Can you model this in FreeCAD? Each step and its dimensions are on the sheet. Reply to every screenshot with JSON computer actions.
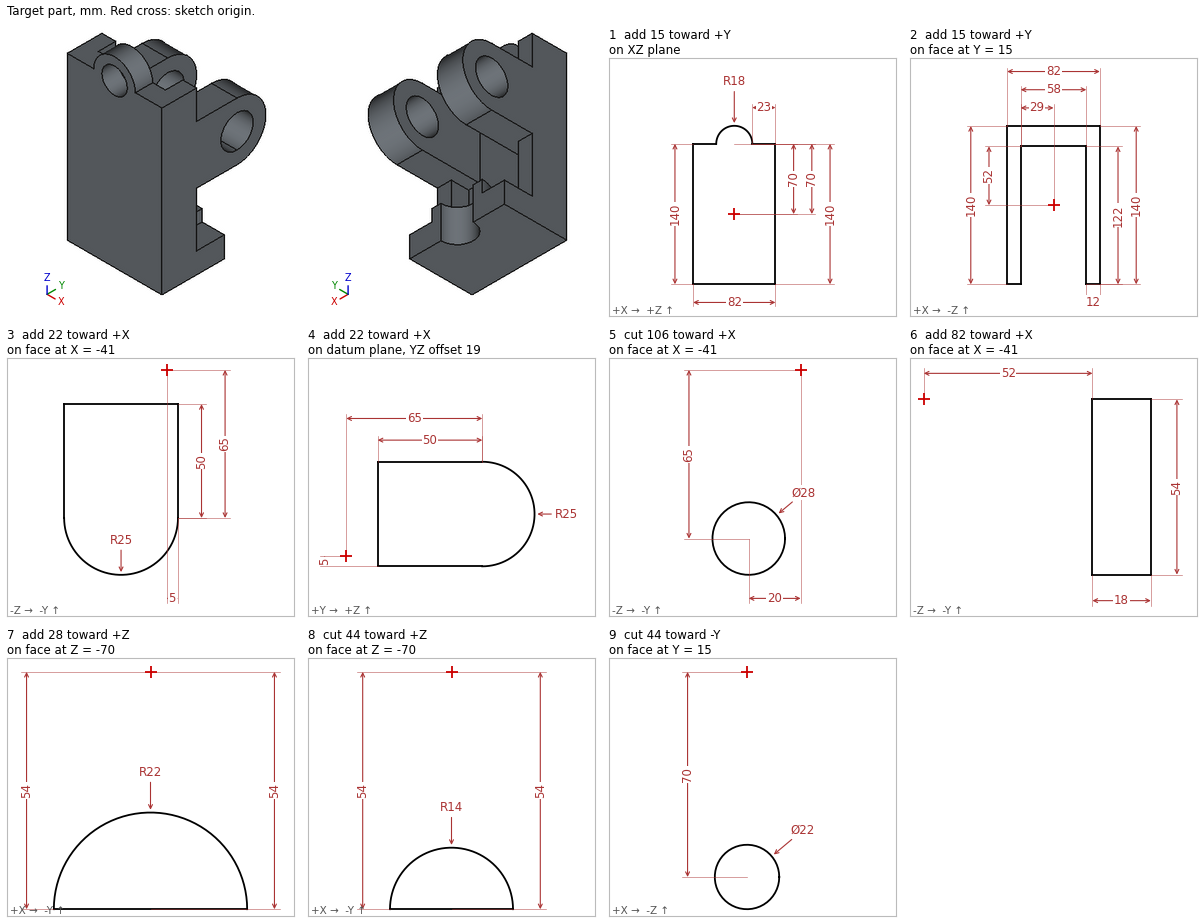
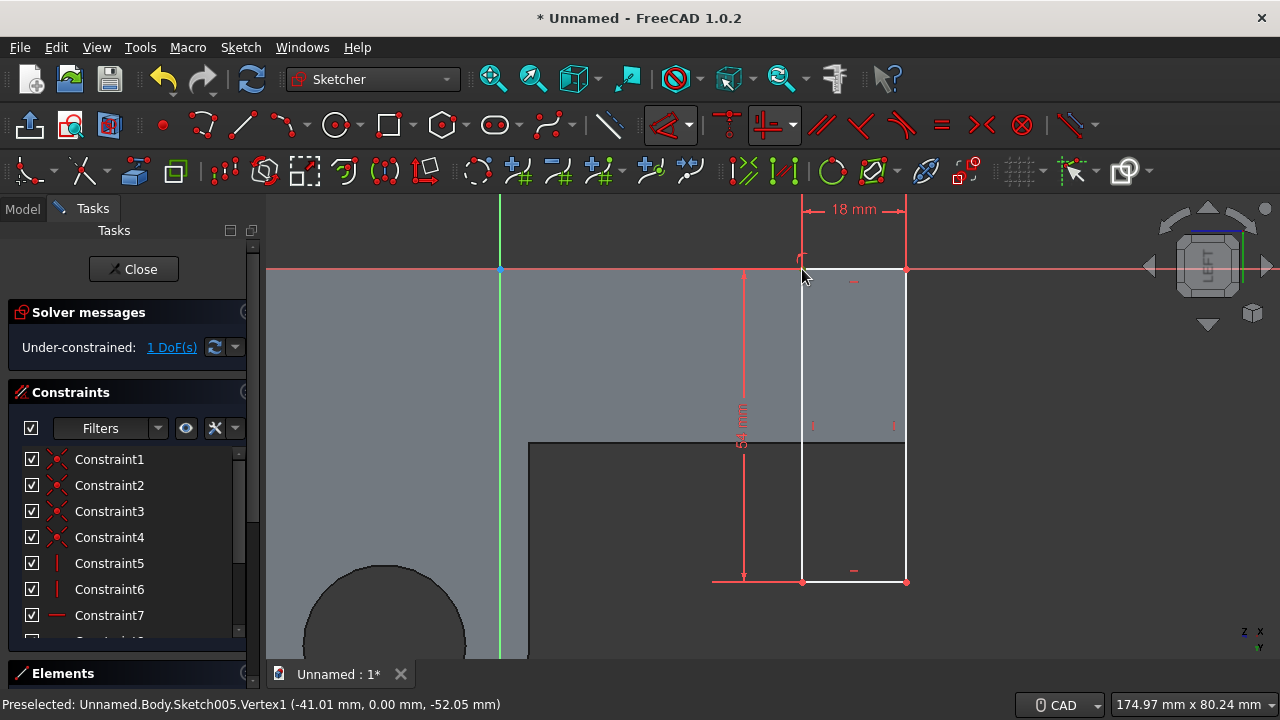
{"action": "key", "text": "l"}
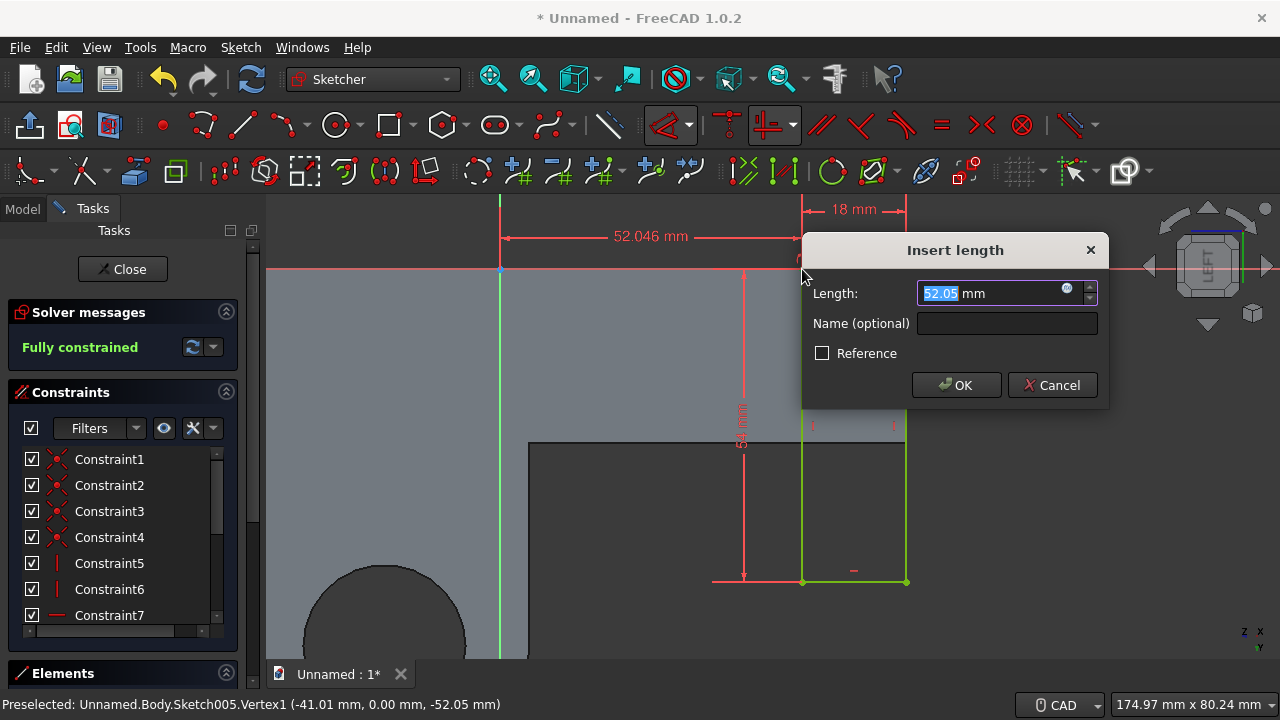
{"action": "type", "text": "52"}
{"action": "key", "text": "Return"}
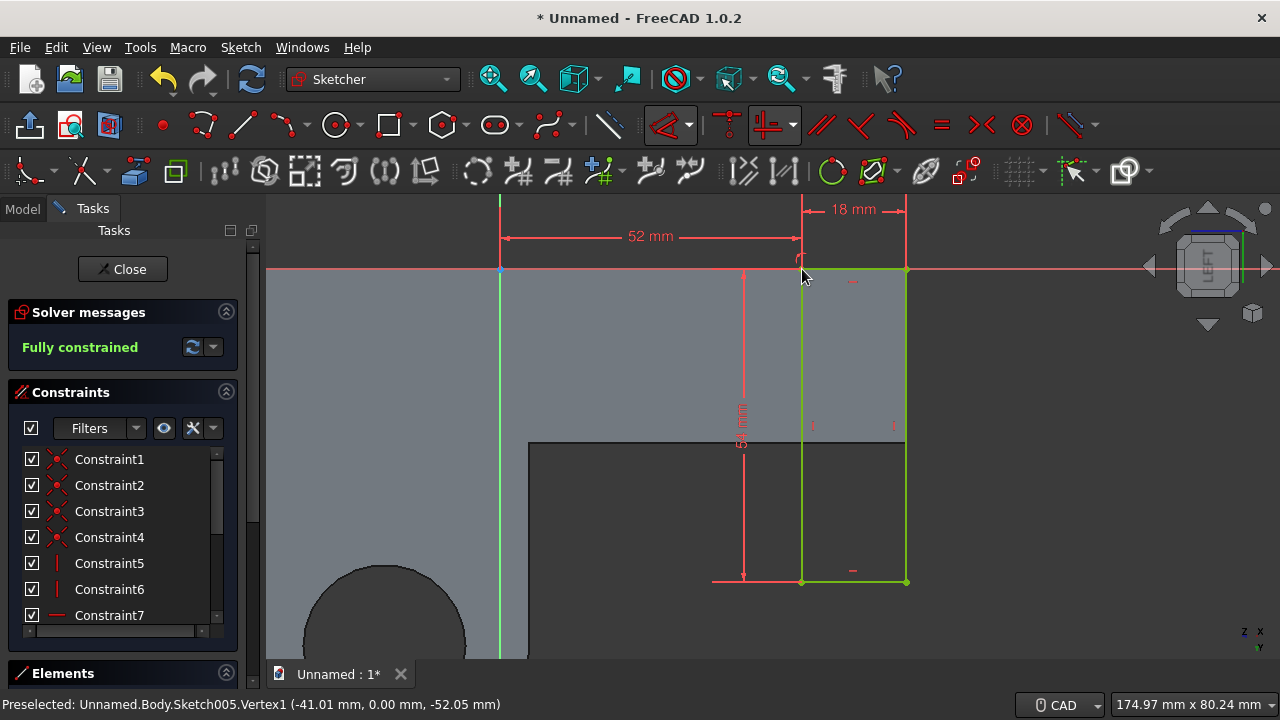
{"action": "left_click", "coordinate": [123, 269]}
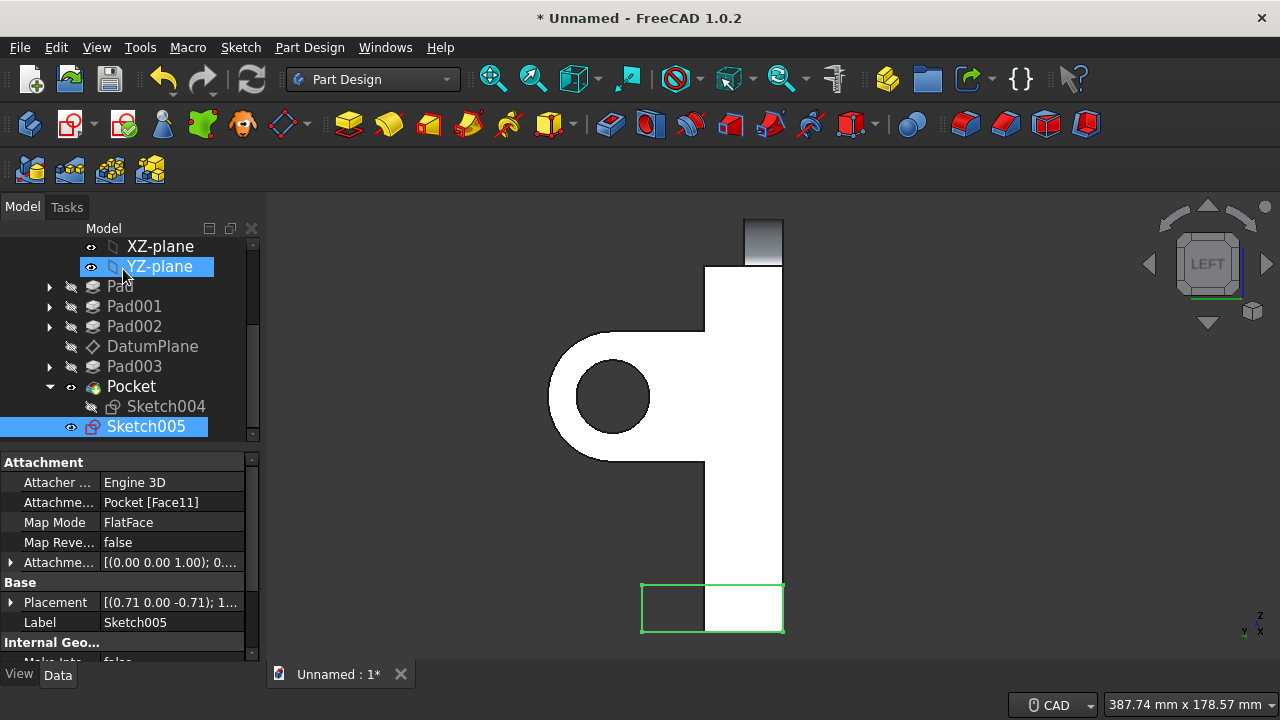
{"action": "left_click", "coordinate": [350, 124]}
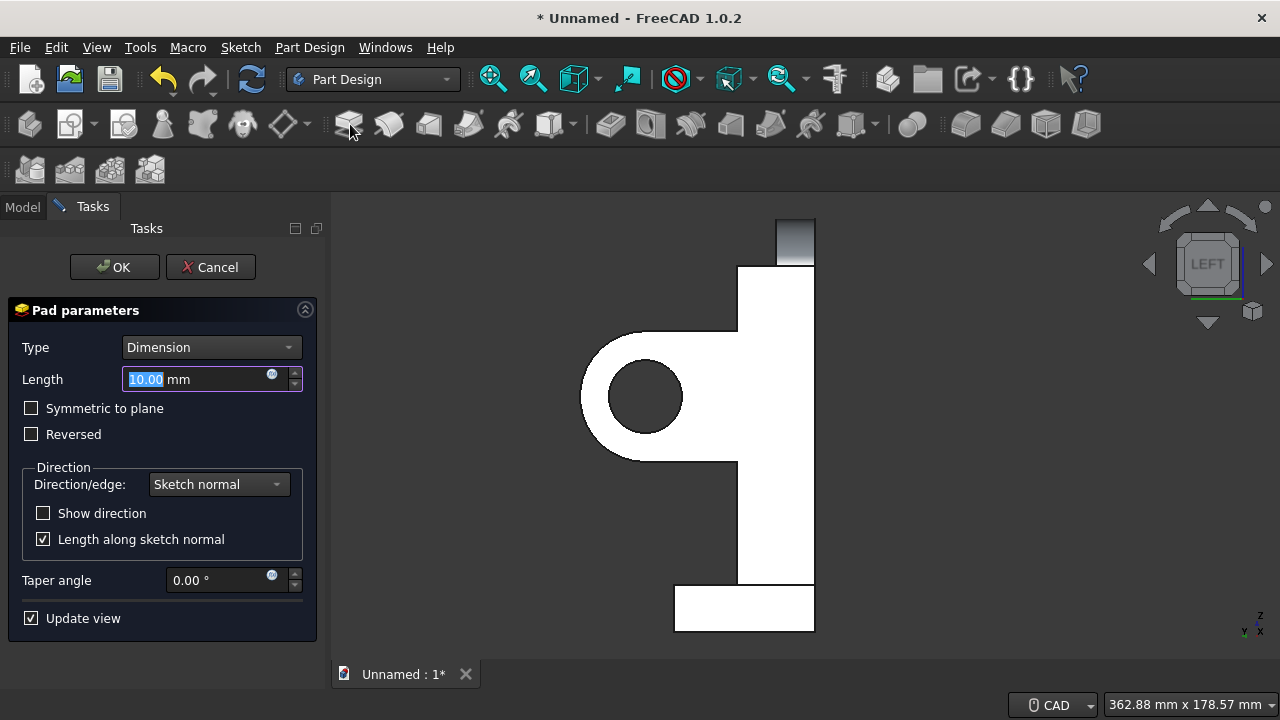
{"action": "type", "text": "82"}
{"action": "key", "text": "Tab"}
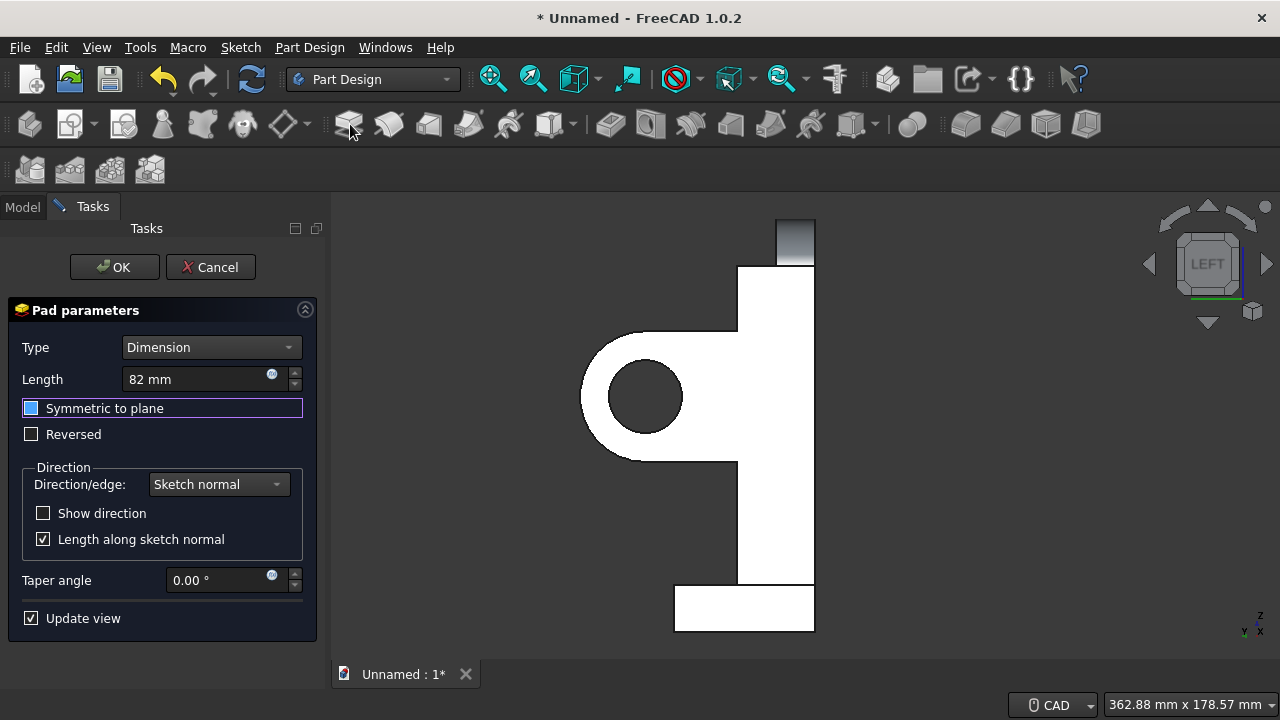
{"action": "left_click", "coordinate": [30, 434]}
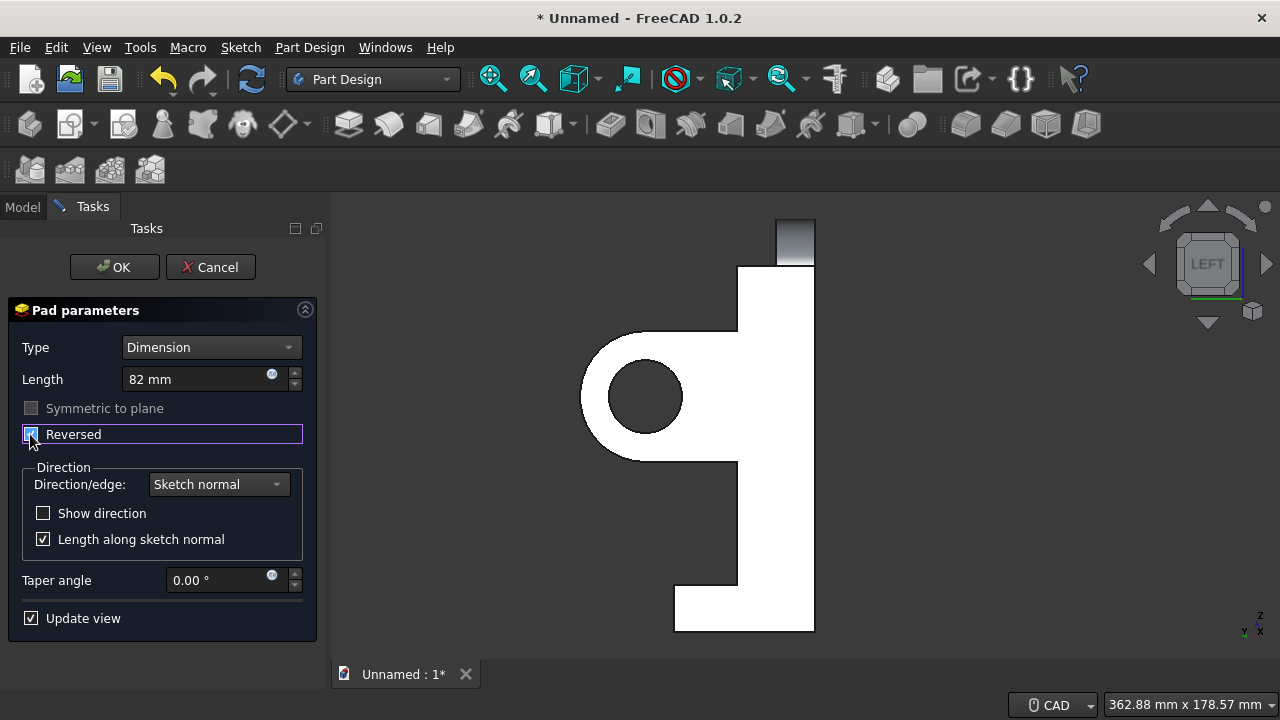
{"action": "left_click", "coordinate": [115, 267]}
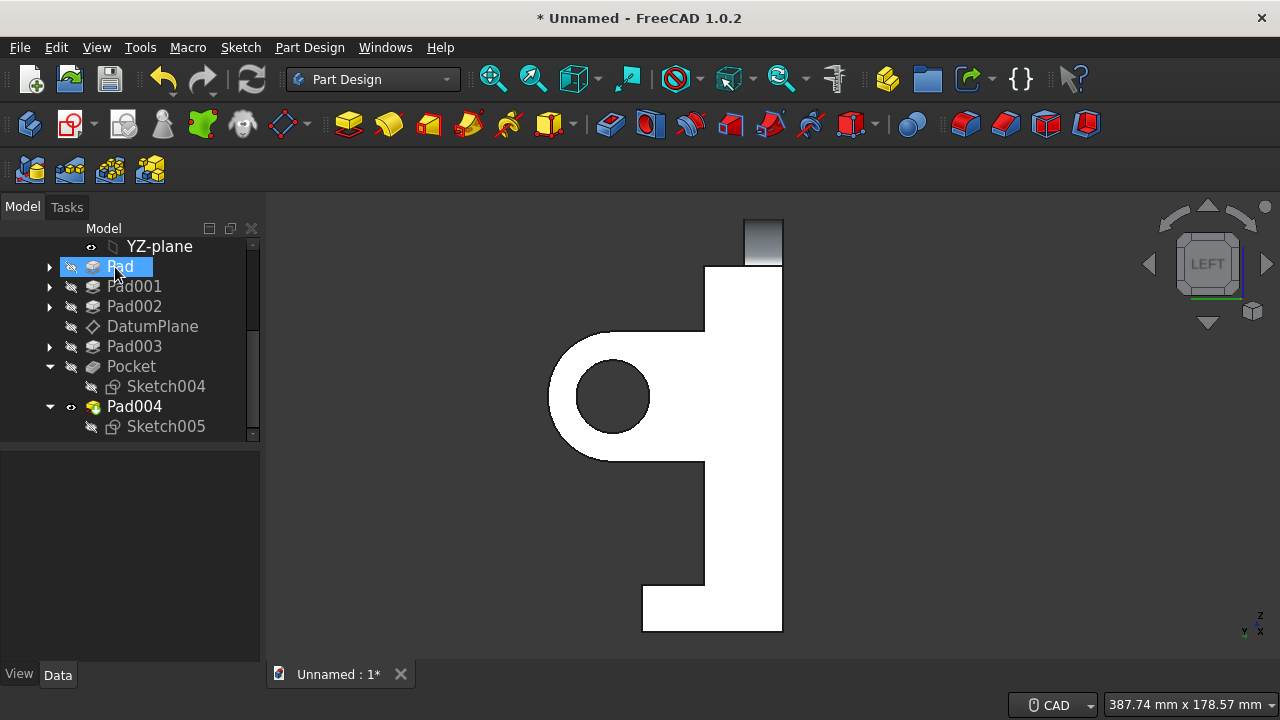
{"action": "key", "text": "5"}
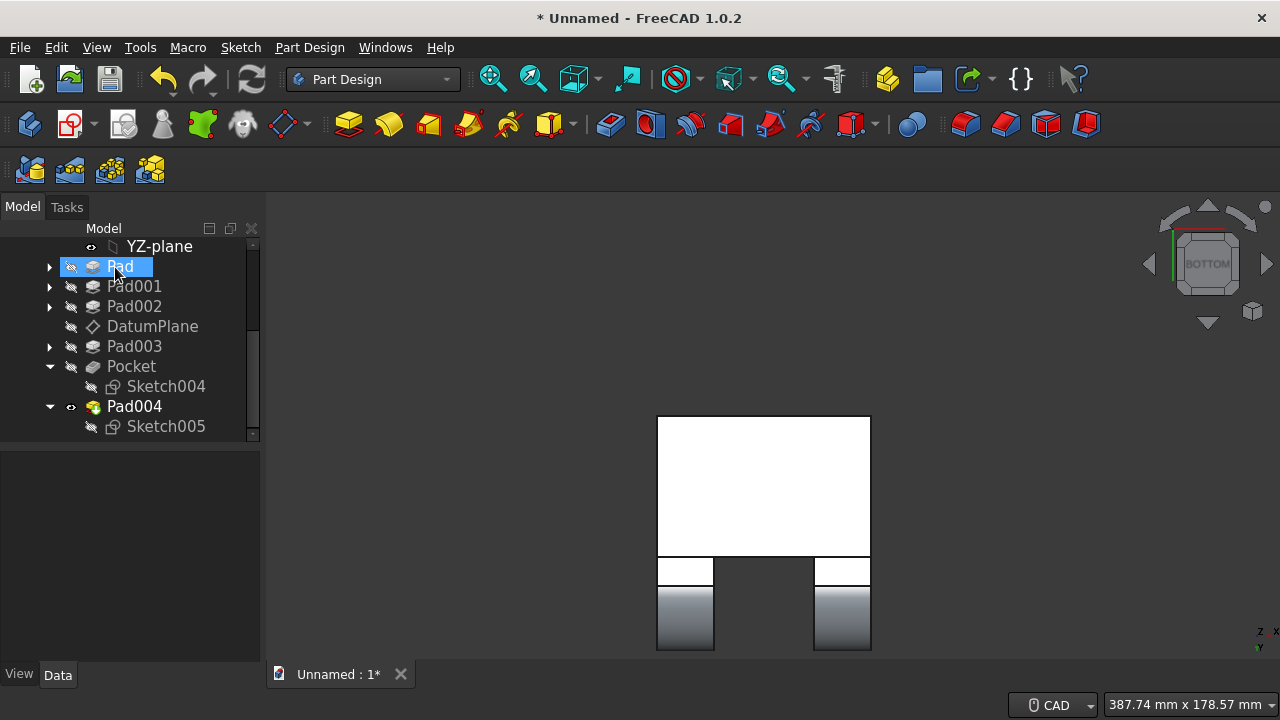
{"action": "left_click", "coordinate": [795, 485]}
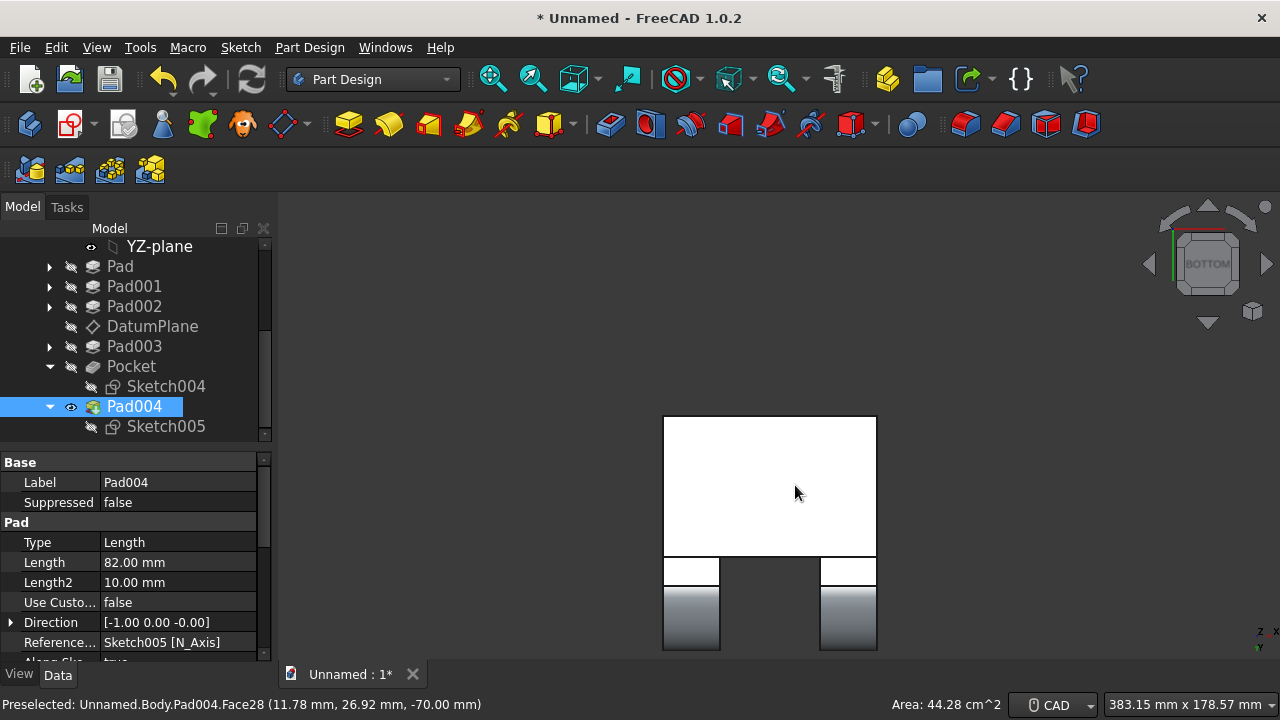
{"action": "left_click", "coordinate": [70, 124]}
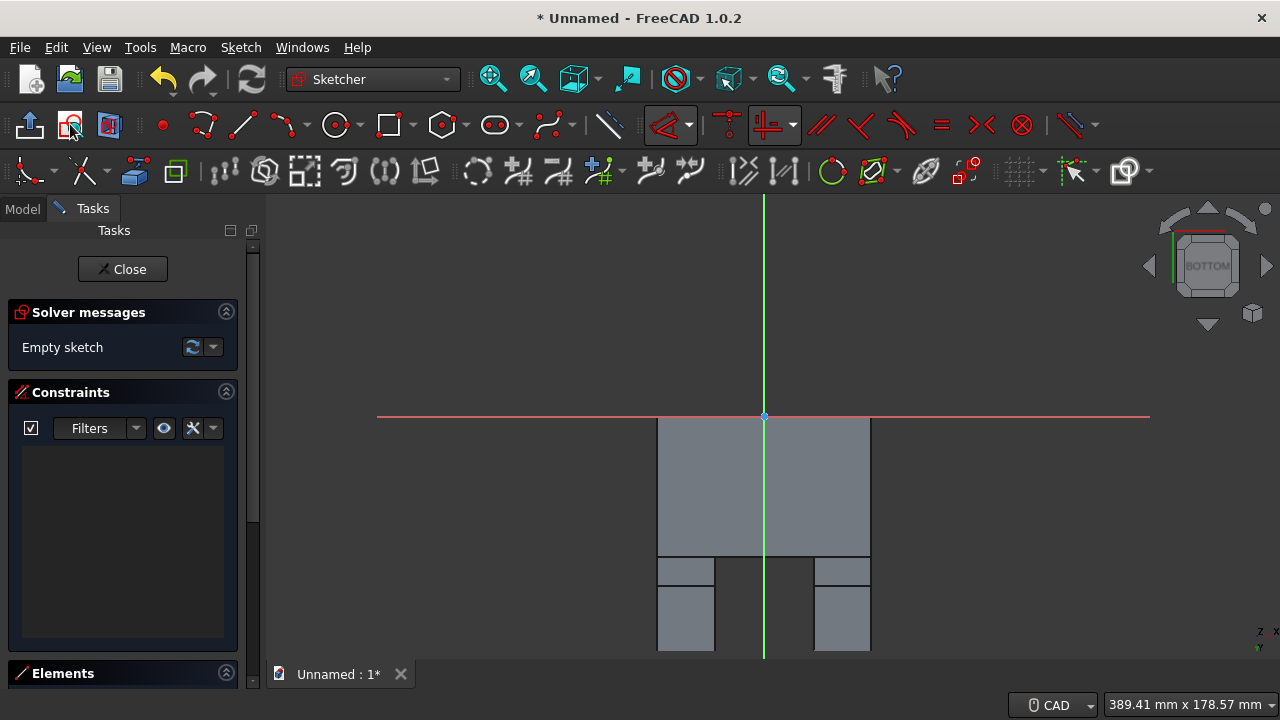
{"action": "scroll", "coordinate": [813, 536], "scroll_direction": "up", "scroll_amount": 4}